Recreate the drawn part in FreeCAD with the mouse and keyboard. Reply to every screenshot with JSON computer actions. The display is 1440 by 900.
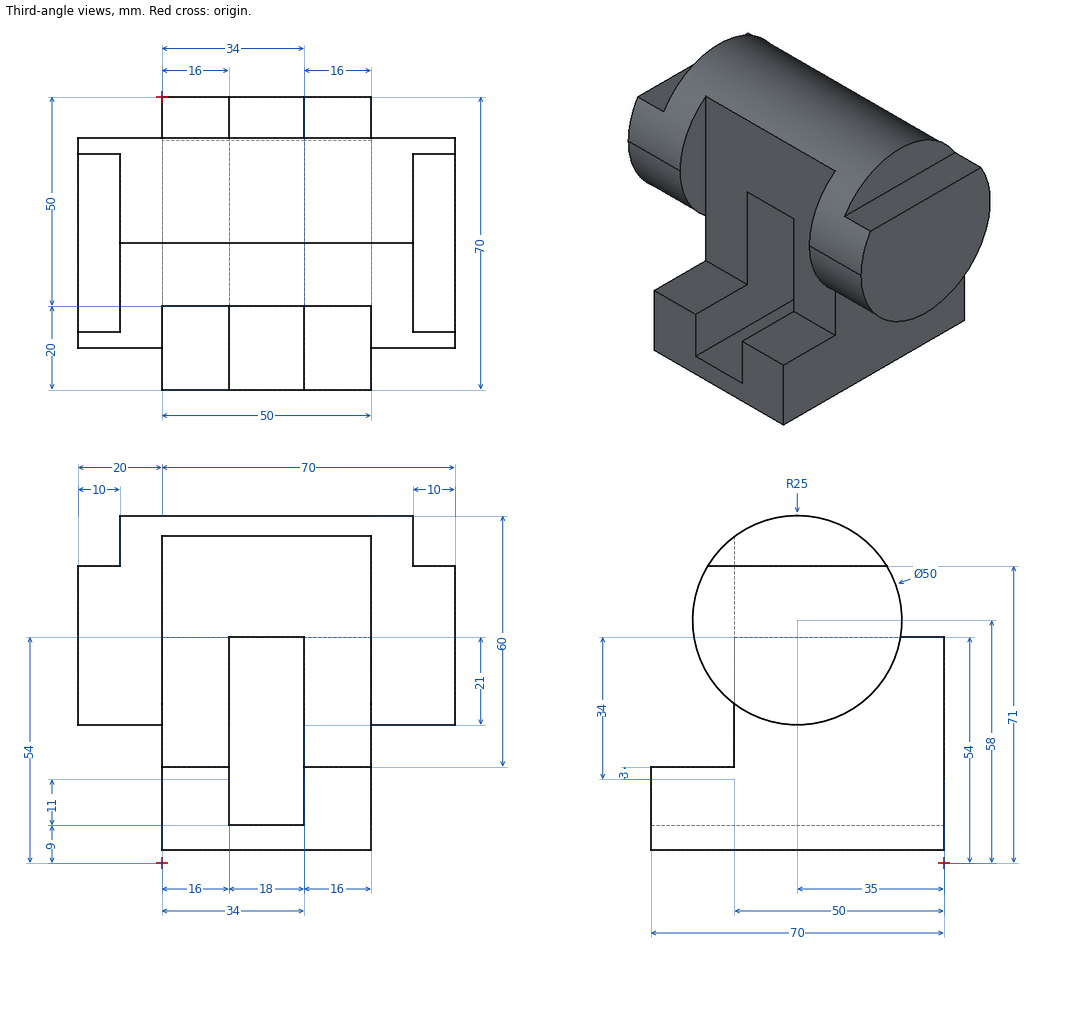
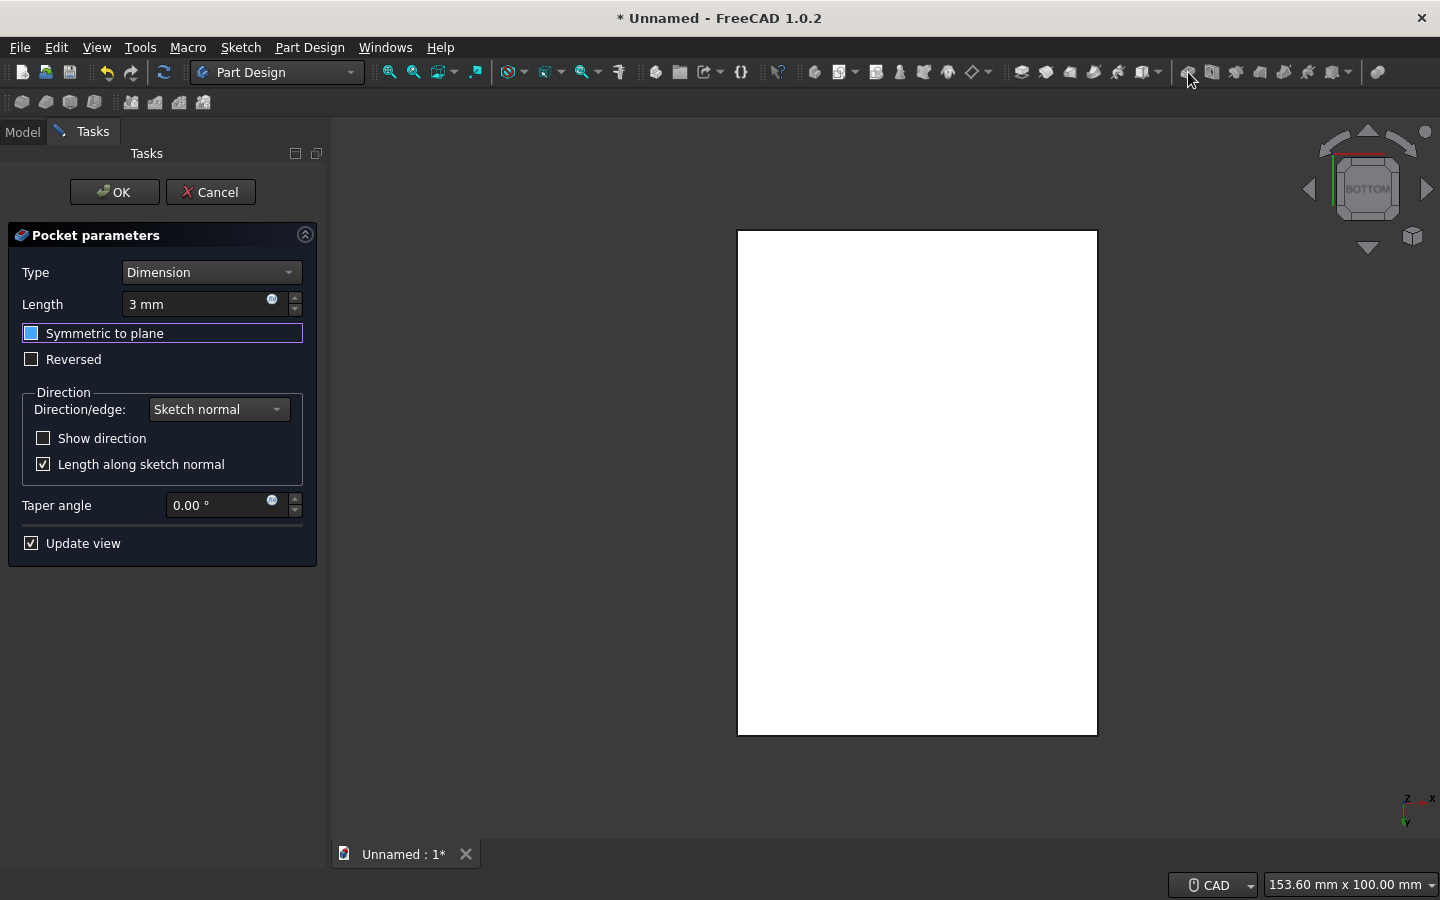
{"action": "left_click", "coordinate": [115, 192]}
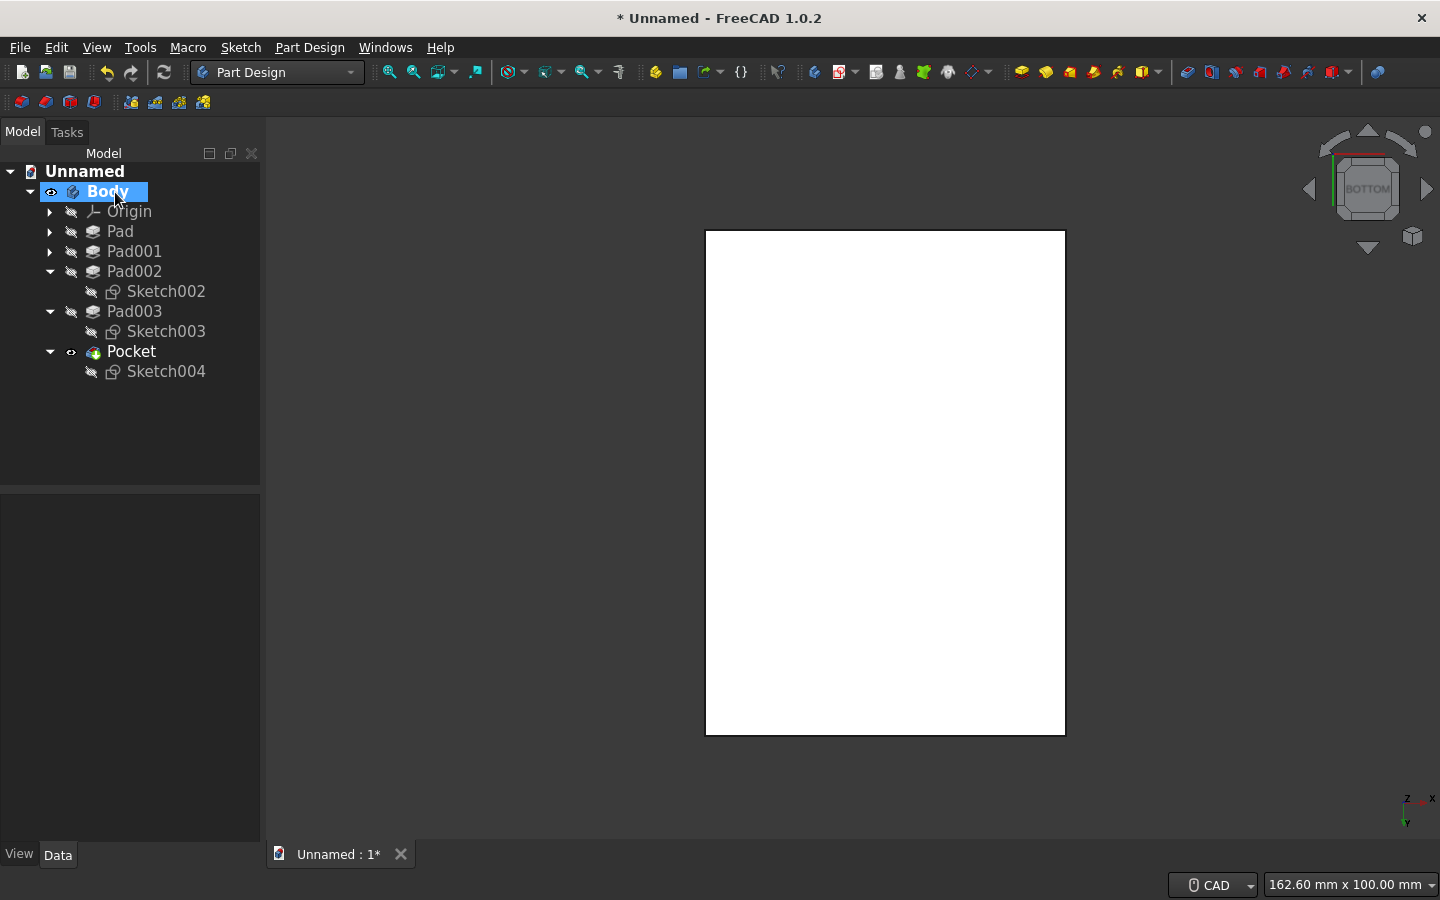
{"action": "key", "text": "0"}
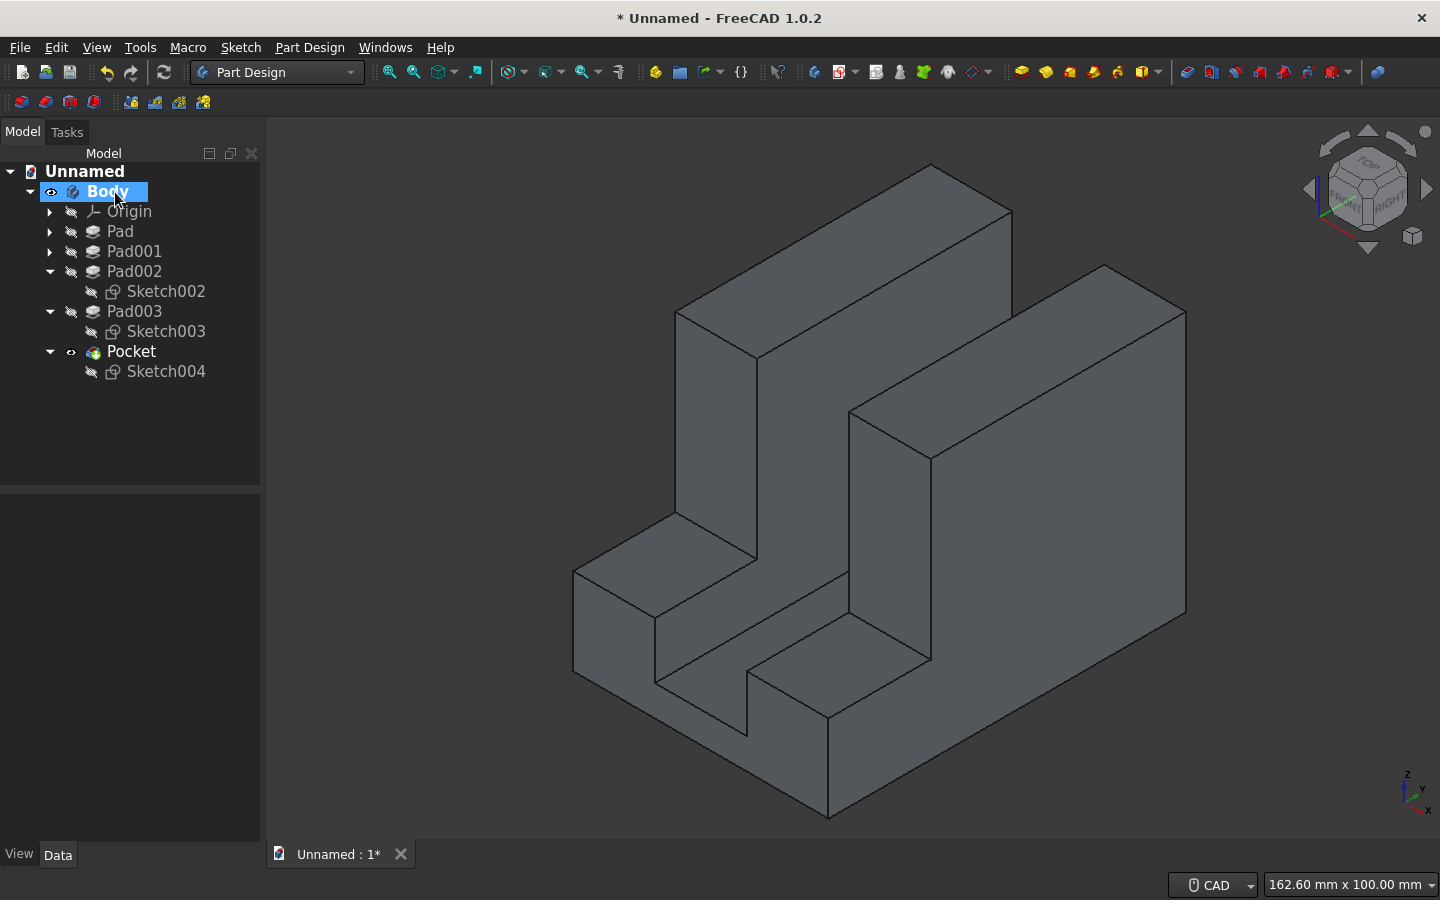
{"action": "left_click", "coordinate": [665, 564]}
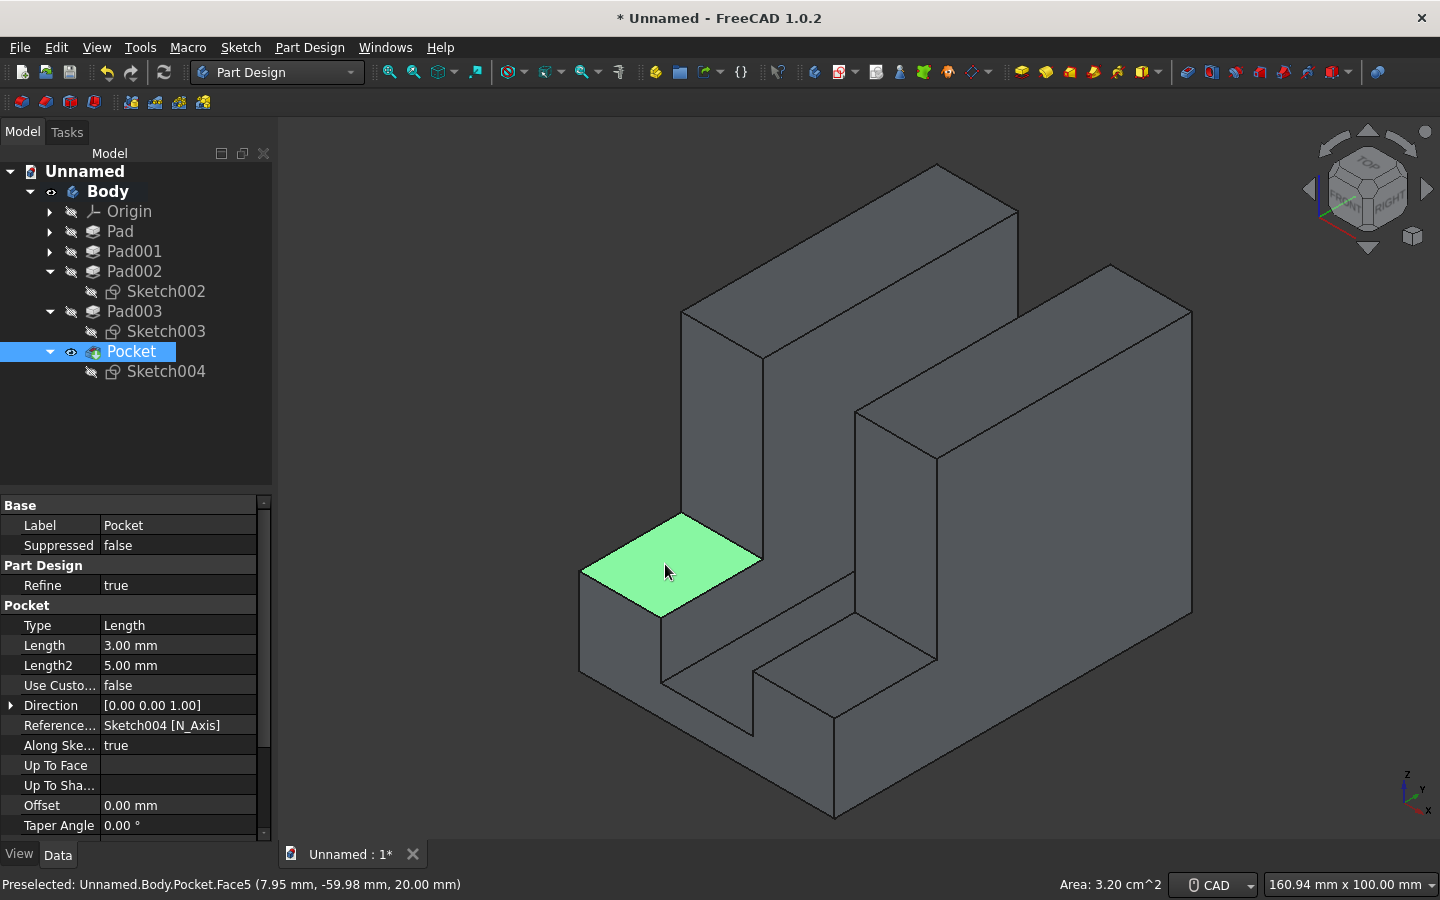
{"action": "left_click", "coordinate": [840, 72]}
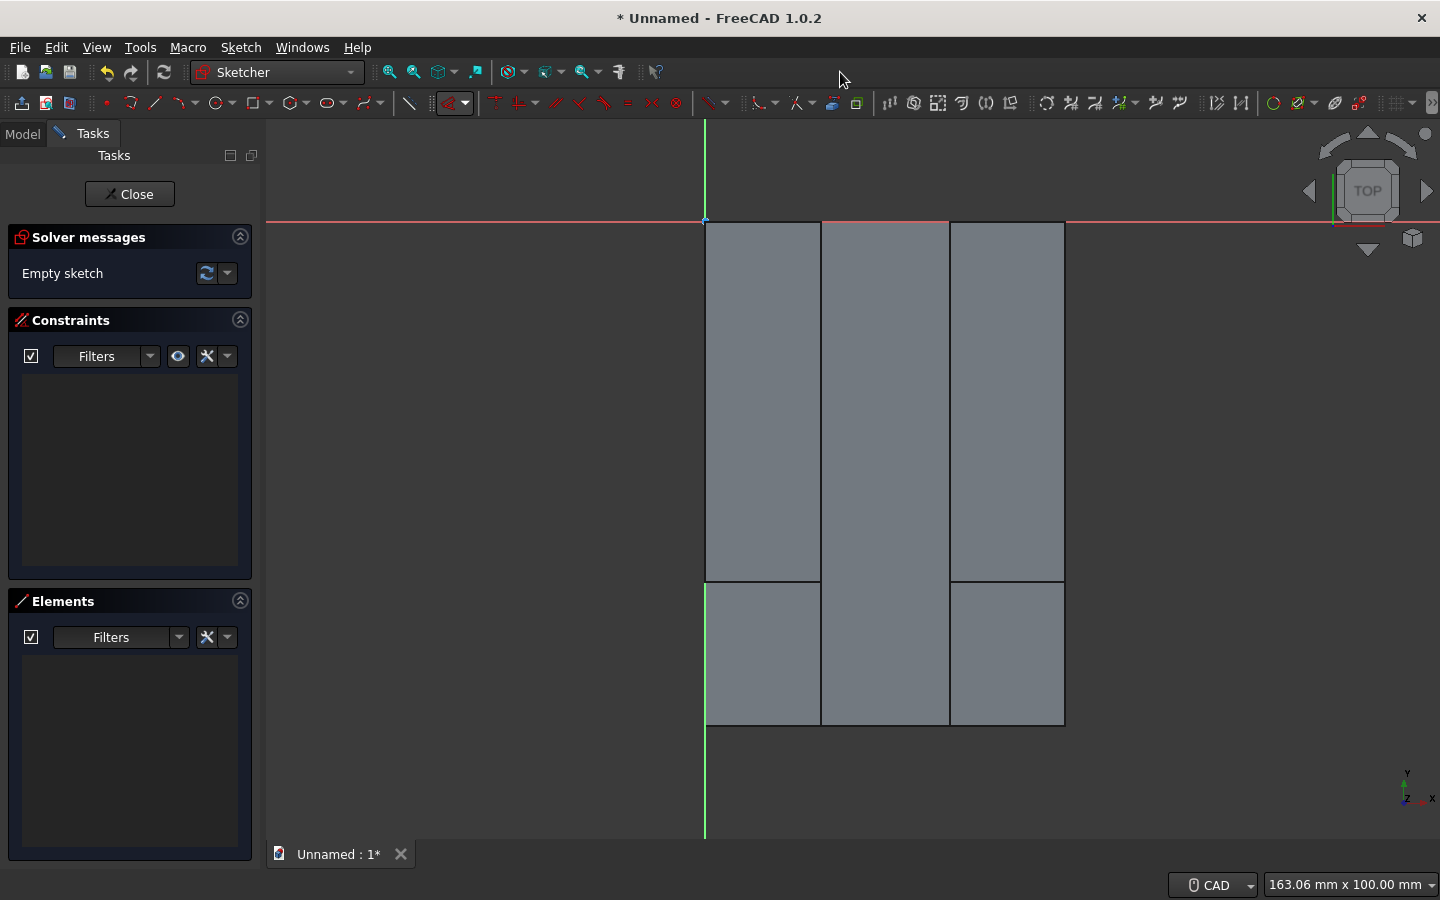
{"action": "left_click", "coordinate": [254, 104]}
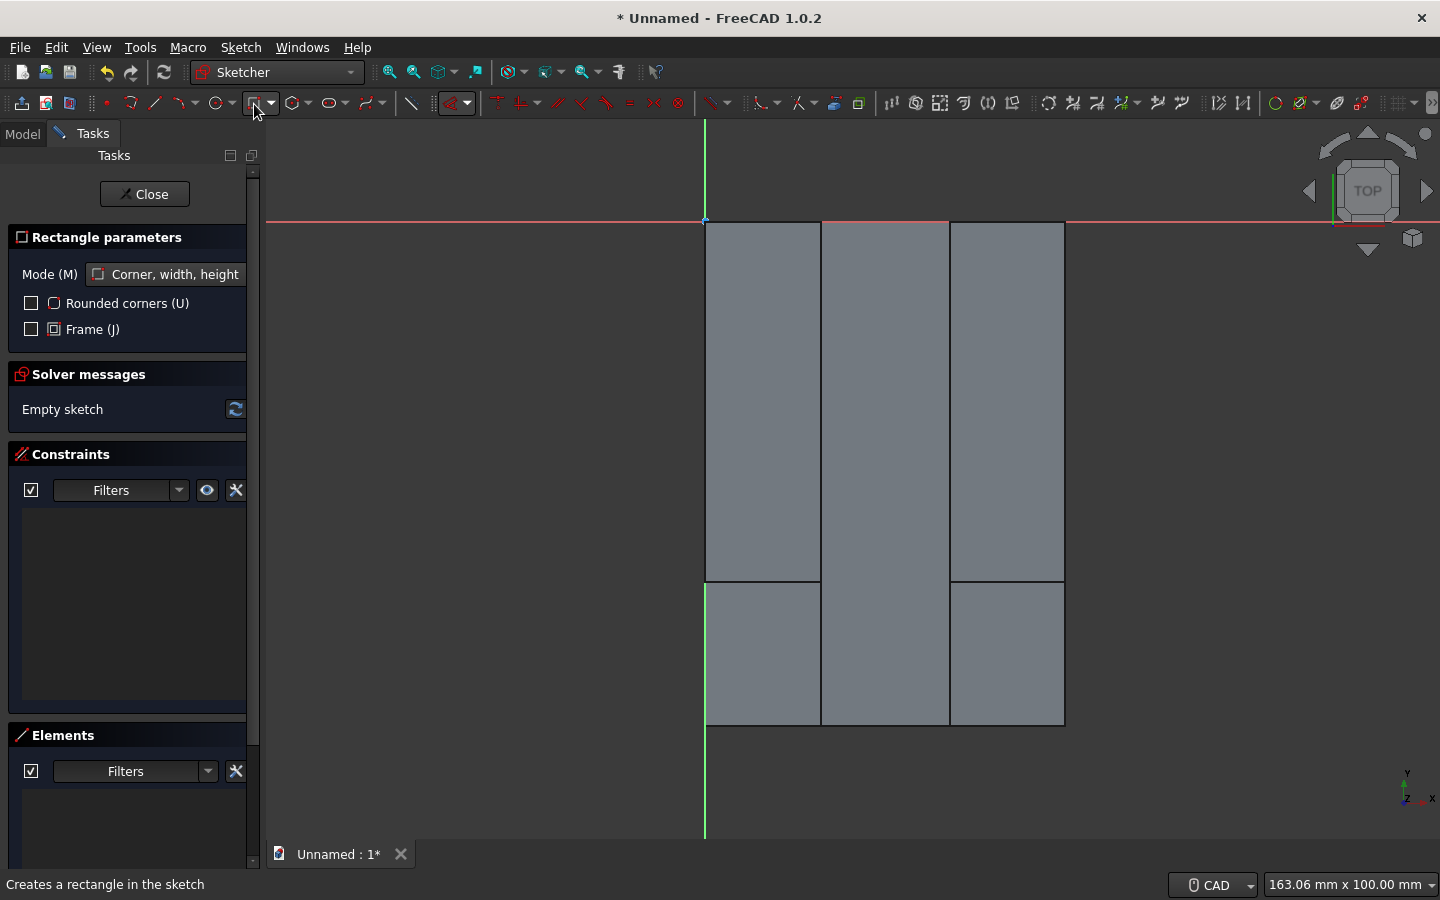
{"action": "left_click", "coordinate": [705, 582]}
{"action": "mouse_move", "coordinate": [821, 726]}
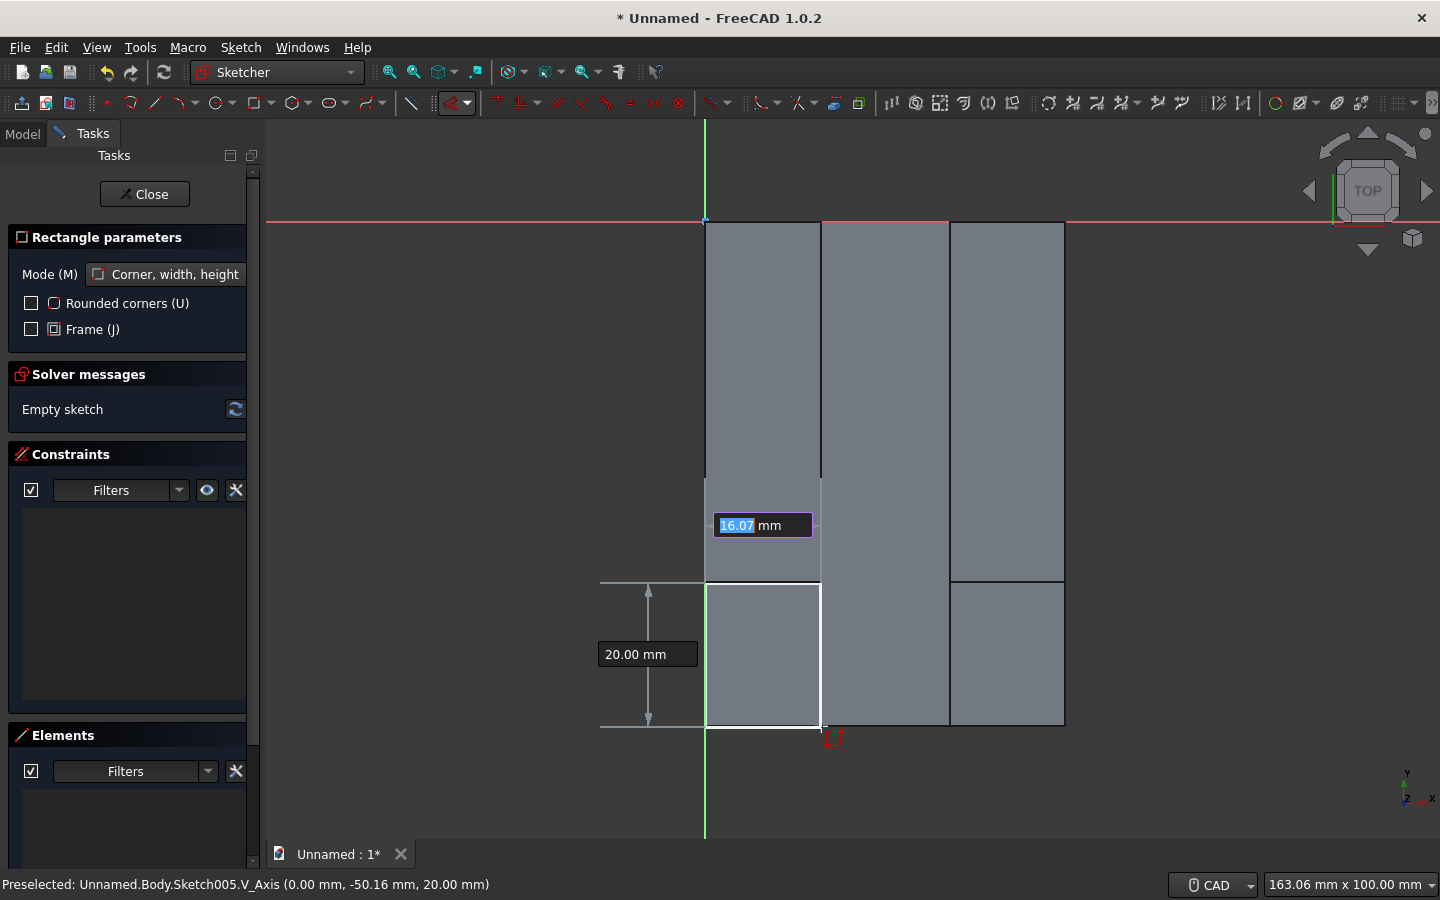
{"action": "type", "text": "16"}
{"action": "key", "text": "Tab"}
{"action": "type", "text": "20"}
{"action": "key", "text": "Return"}